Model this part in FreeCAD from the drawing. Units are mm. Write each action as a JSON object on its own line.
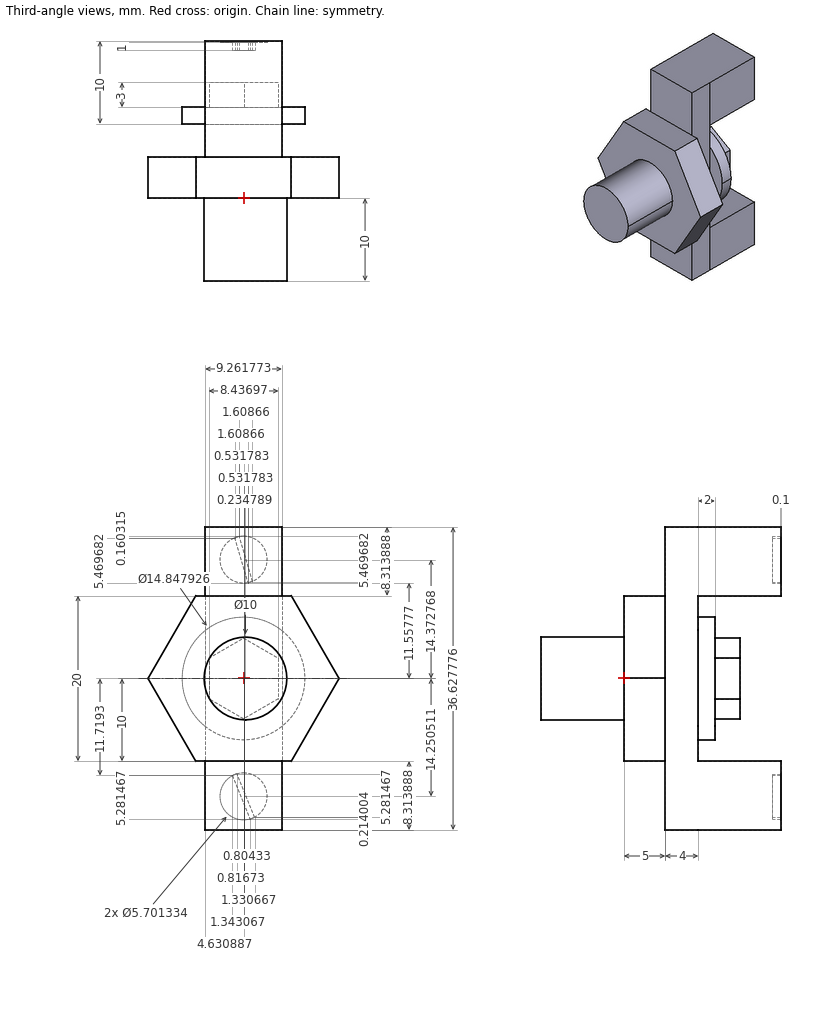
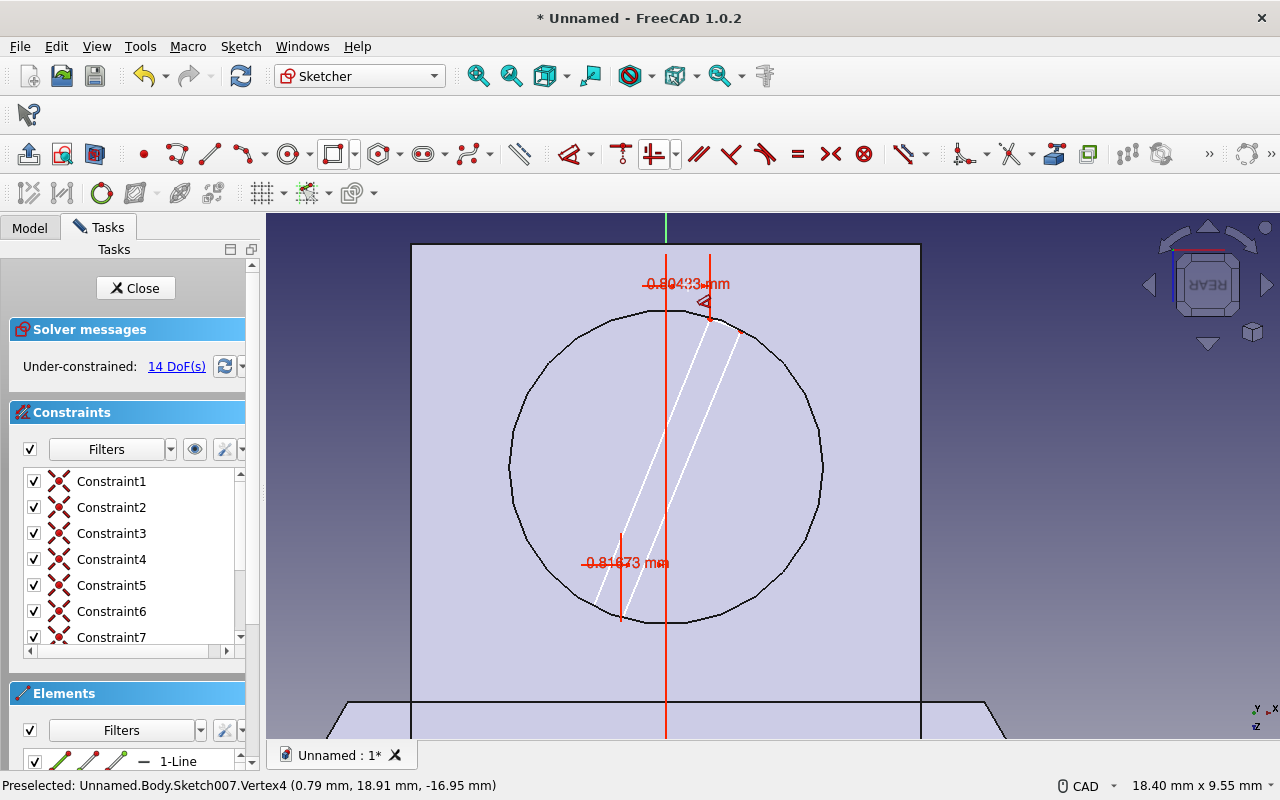
{"action": "left_click", "coordinate": [593, 608]}
{"action": "left_click", "coordinate": [559, 660]}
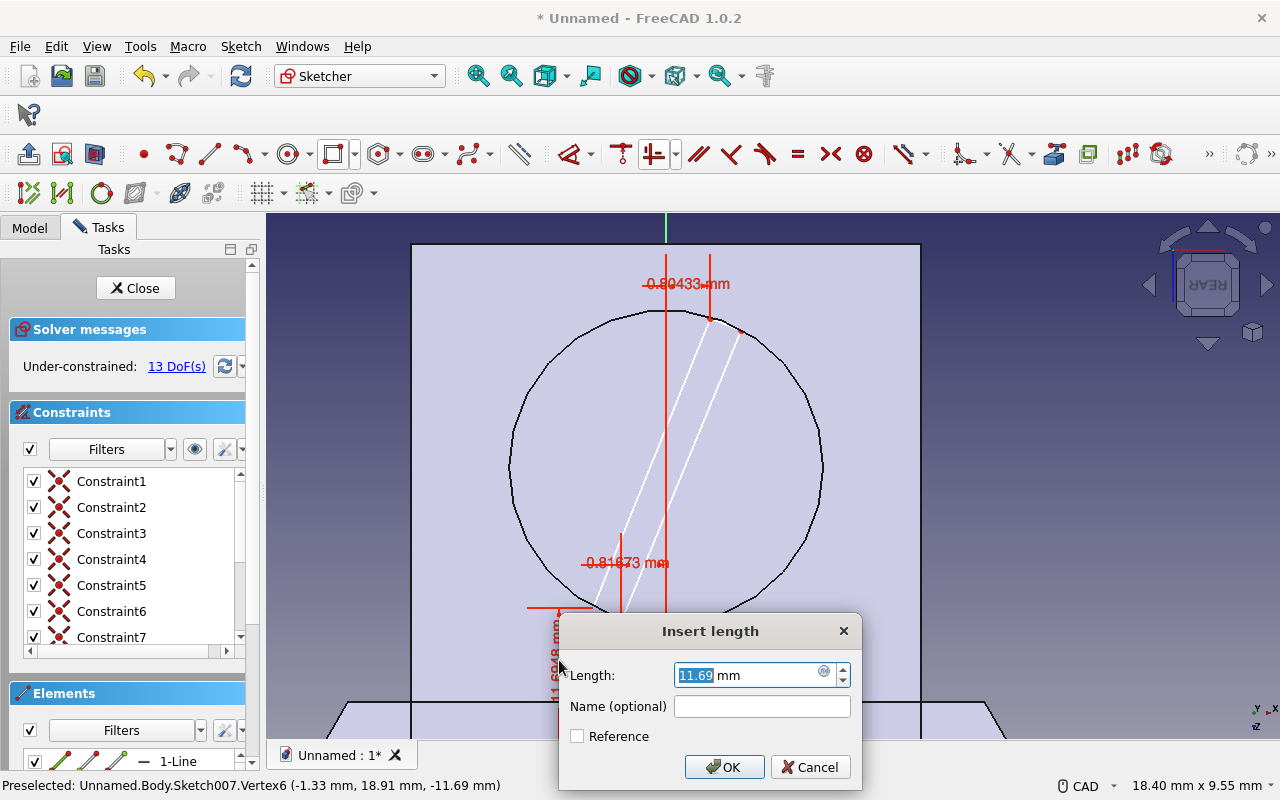
{"action": "type", "text": "11.7193"}
{"action": "key", "text": "Return"}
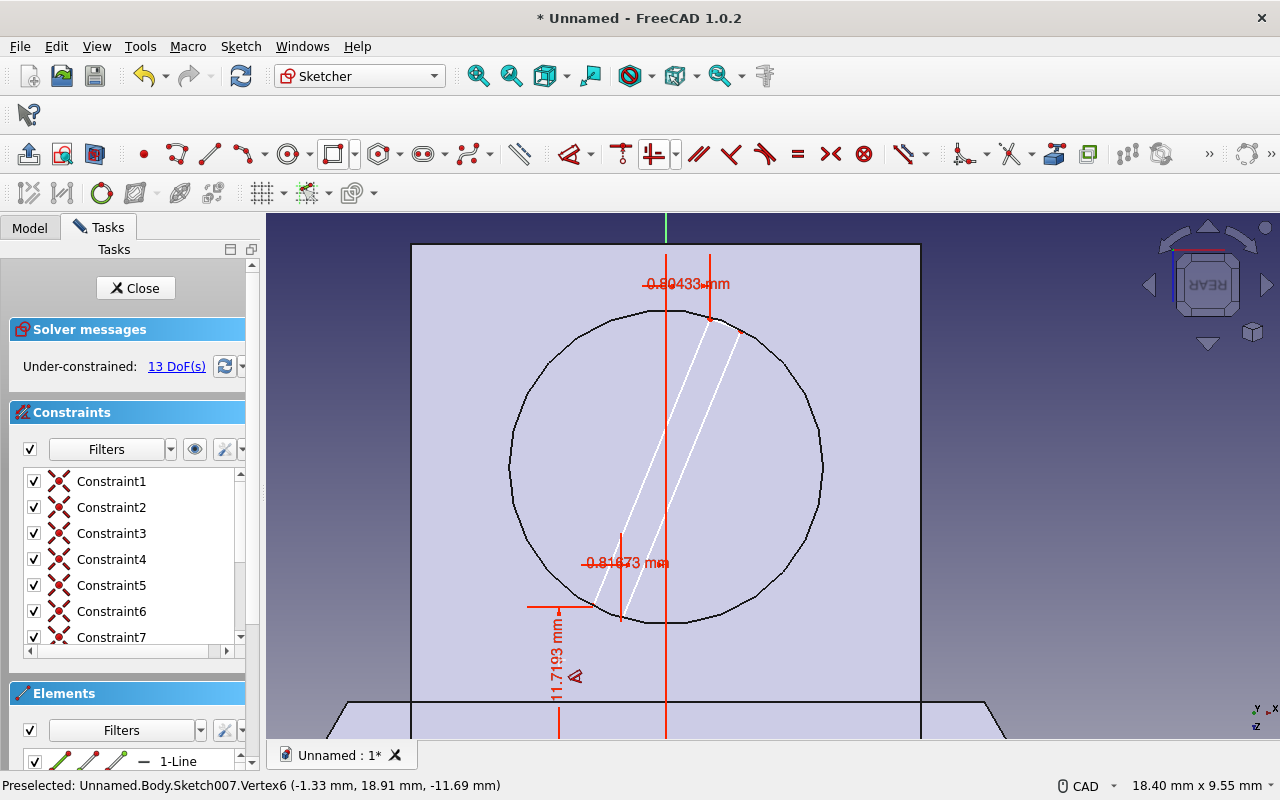
{"action": "scroll", "coordinate": [712, 321], "scroll_direction": "down", "scroll_amount": 9}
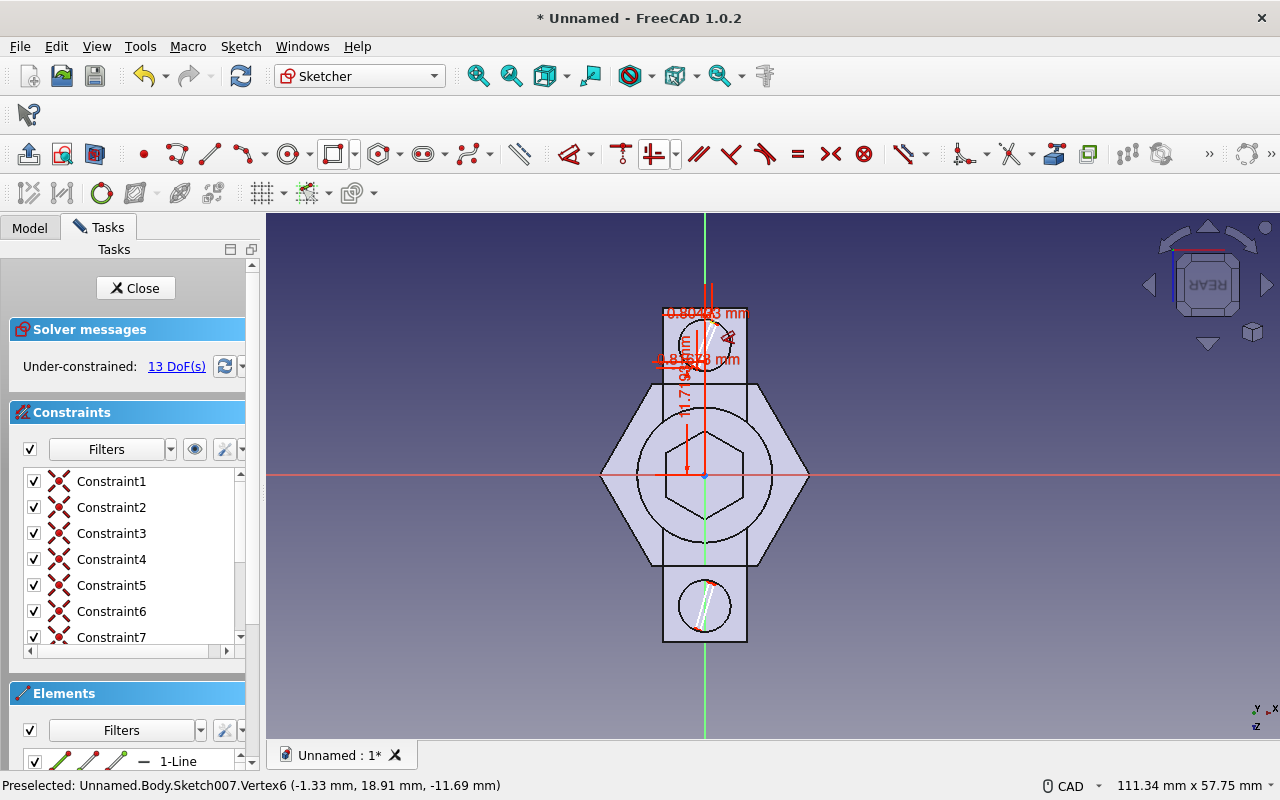
{"action": "scroll", "coordinate": [705, 596], "scroll_direction": "up", "scroll_amount": 5}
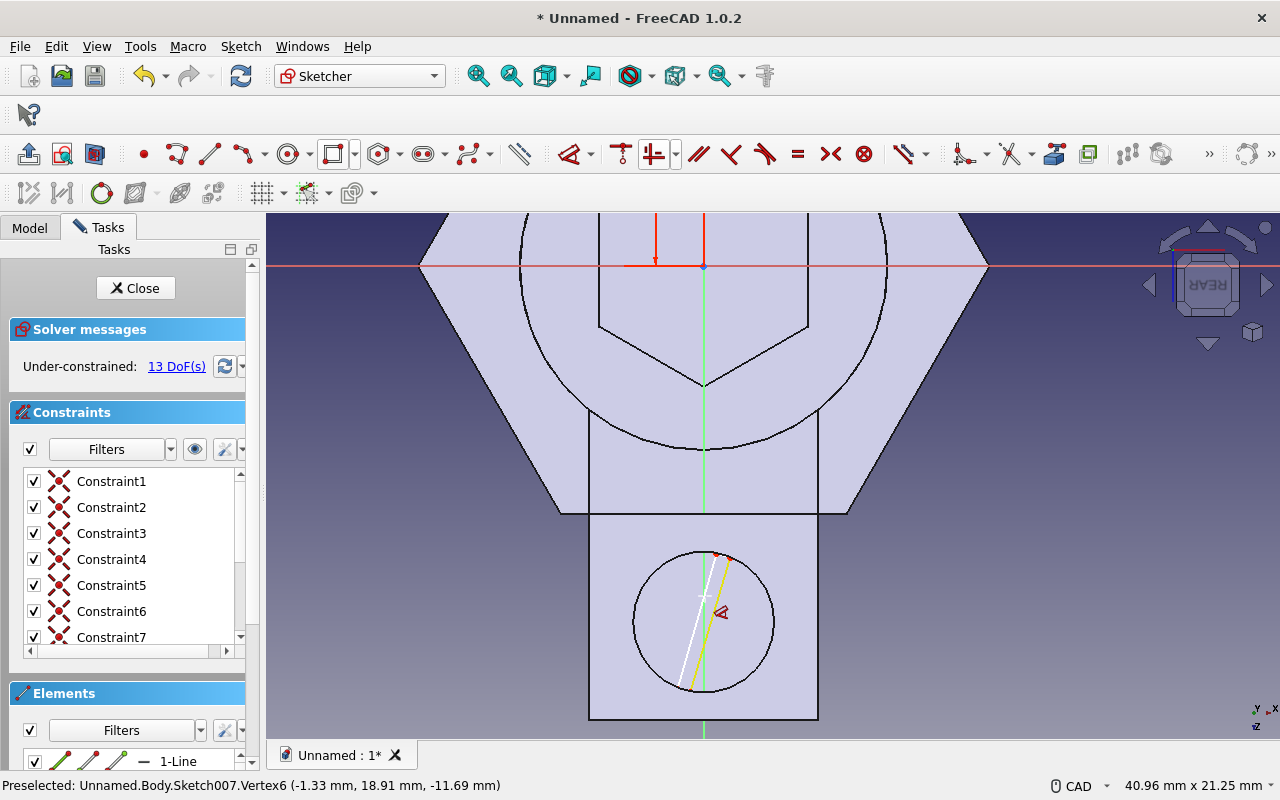
{"action": "left_click", "coordinate": [705, 594]}
{"action": "left_click", "coordinate": [688, 519]}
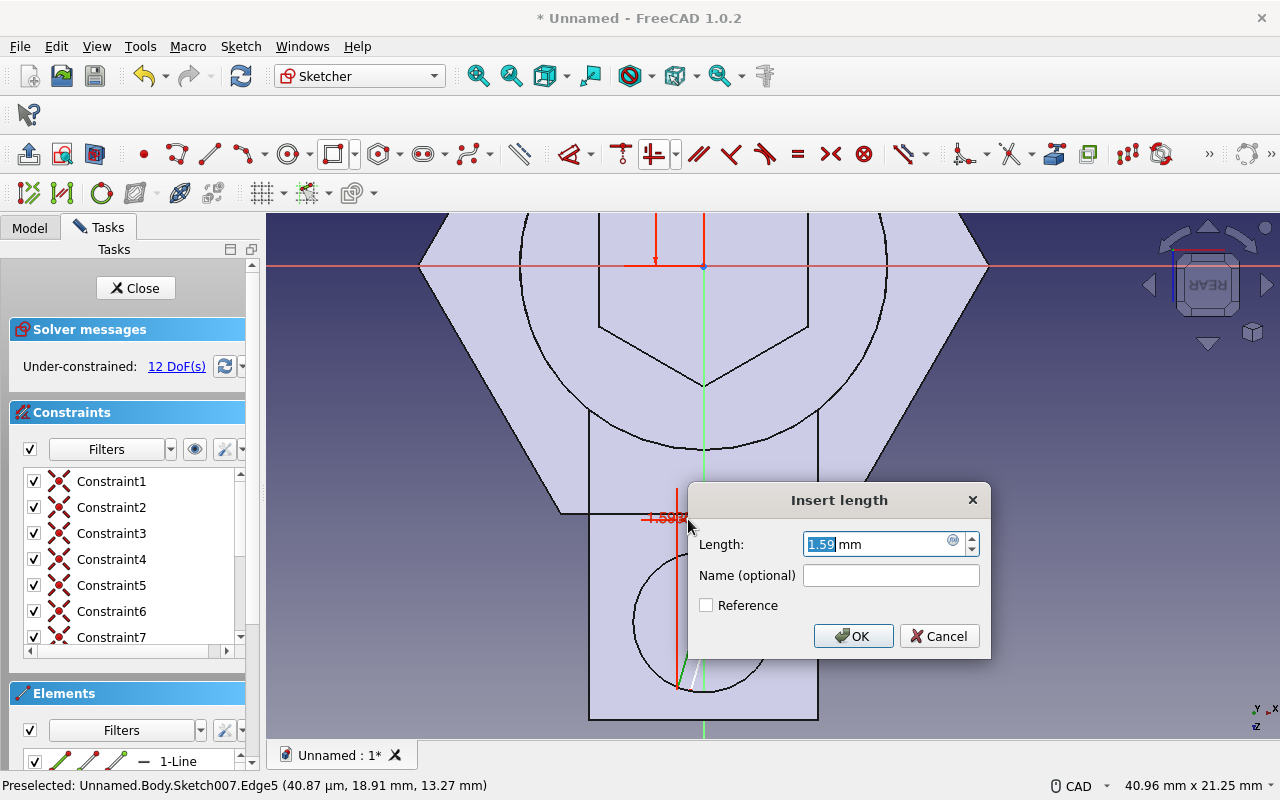
{"action": "type", "text": "1.60866"}
{"action": "key", "text": "Return"}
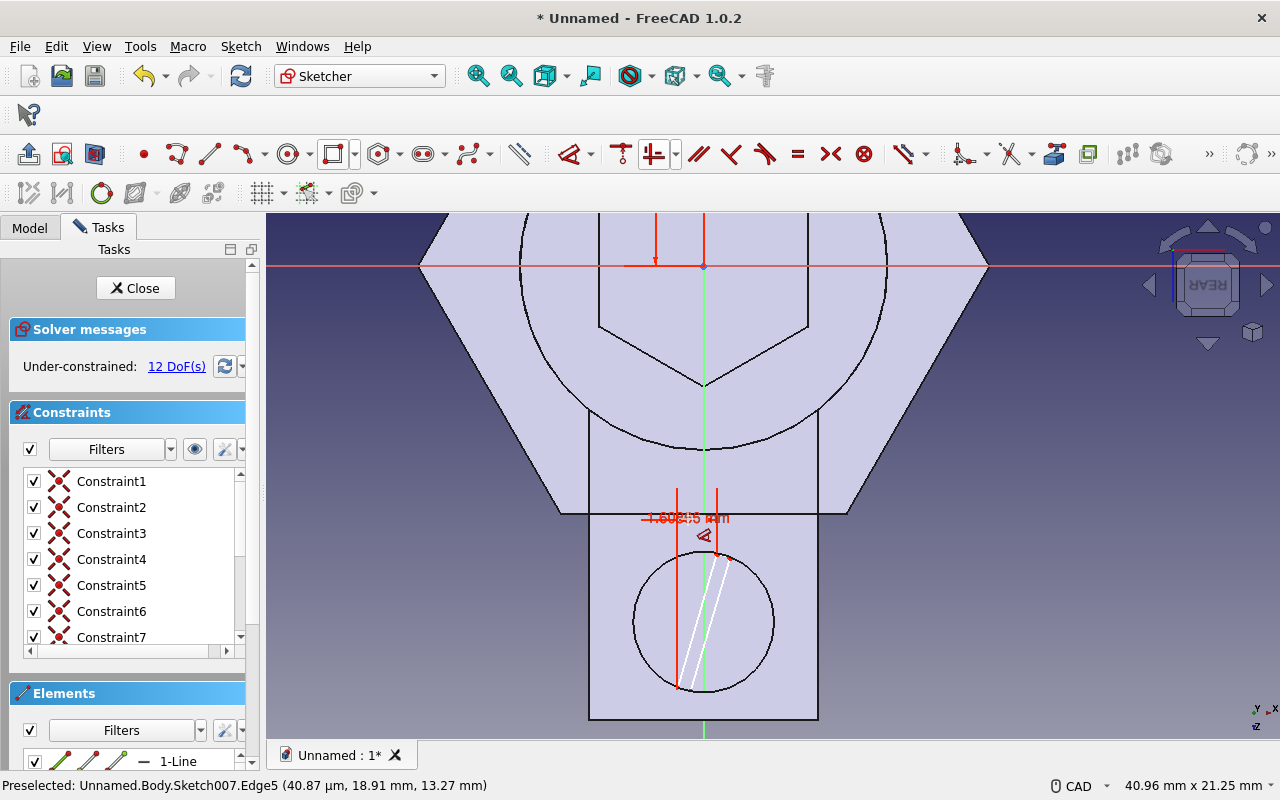
{"action": "left_click", "coordinate": [702, 652]}
{"action": "left_click", "coordinate": [719, 476]}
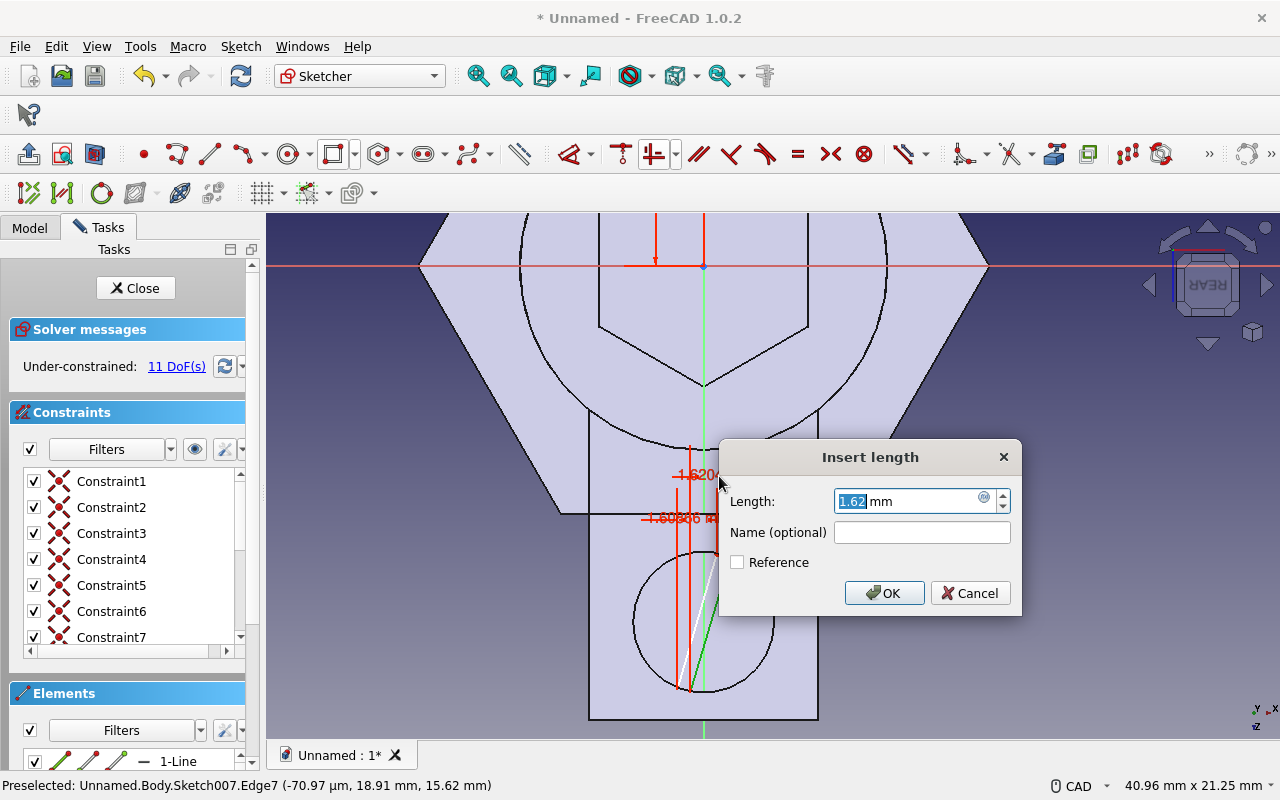
{"action": "type", "text": "1.60866"}
{"action": "key", "text": "Return"}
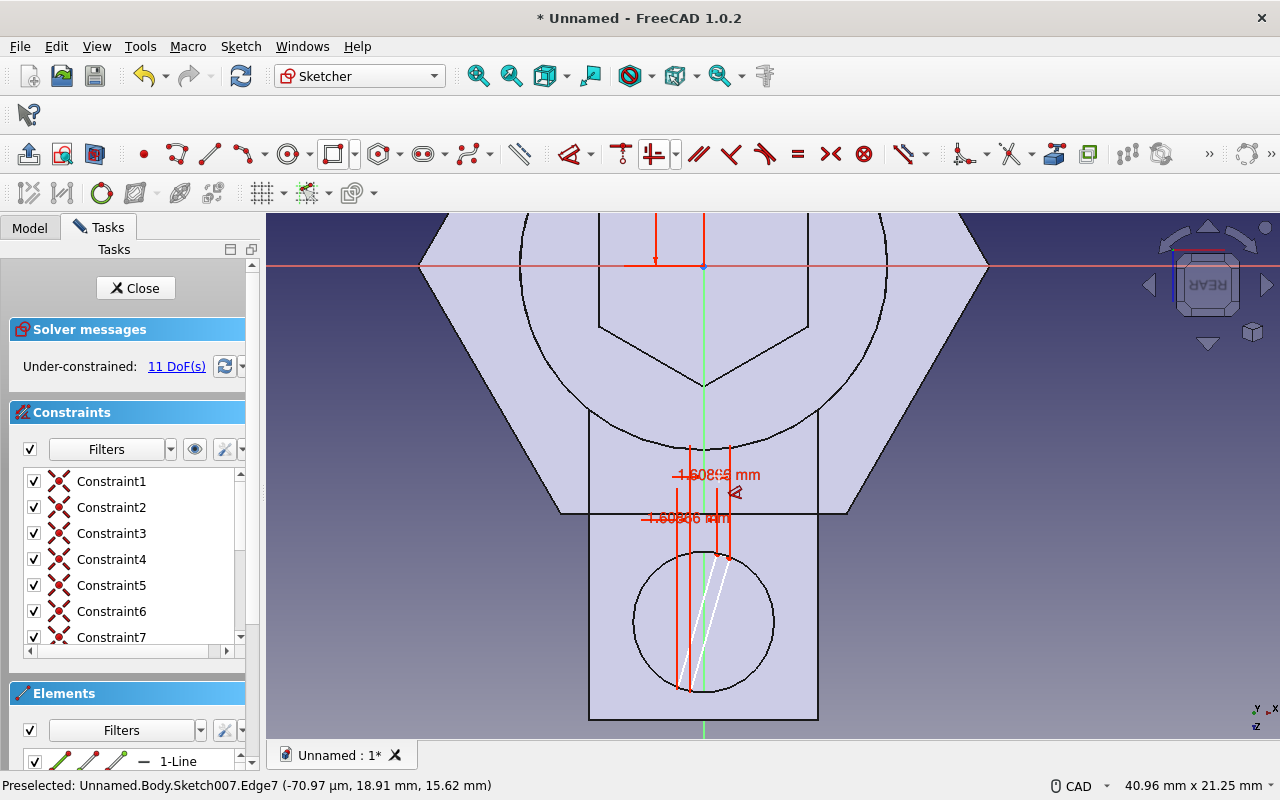
{"action": "scroll", "coordinate": [705, 597], "scroll_direction": "down", "scroll_amount": 5}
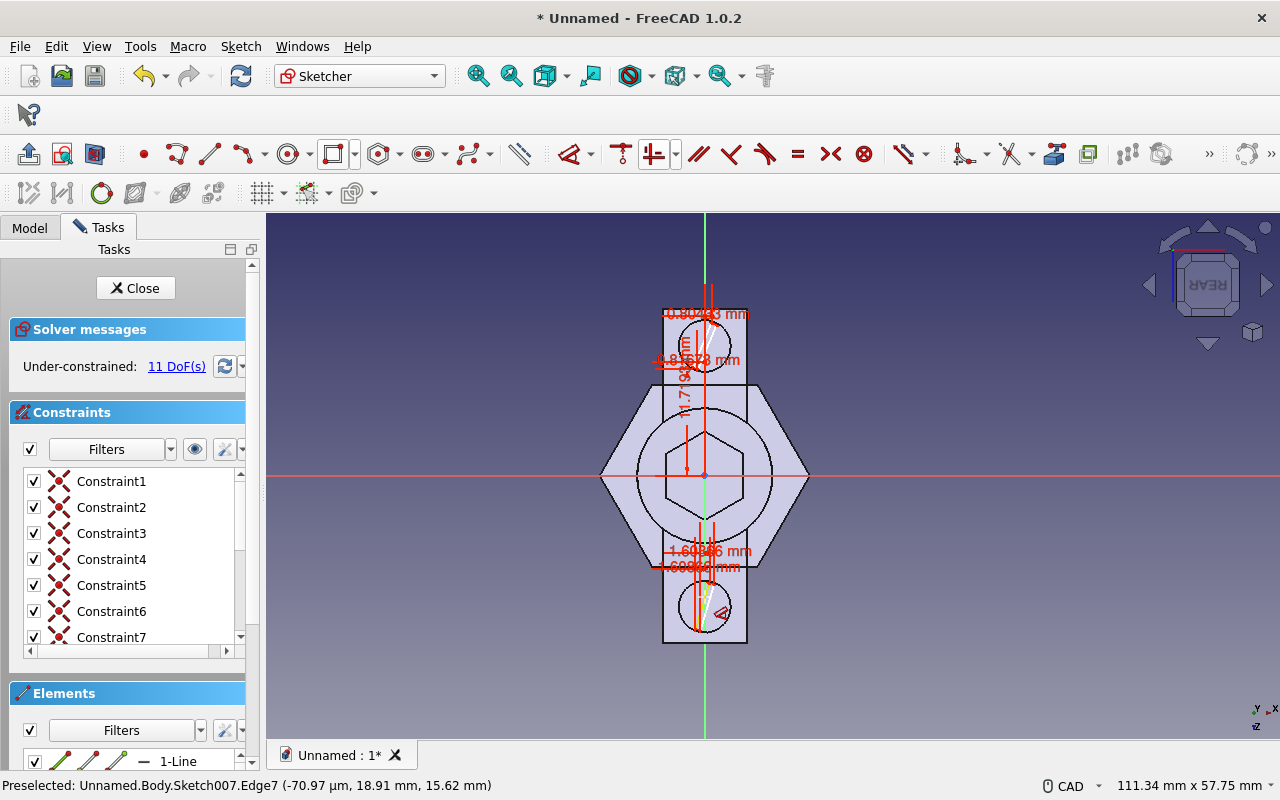
{"action": "scroll", "coordinate": [717, 323], "scroll_direction": "up", "scroll_amount": 6}